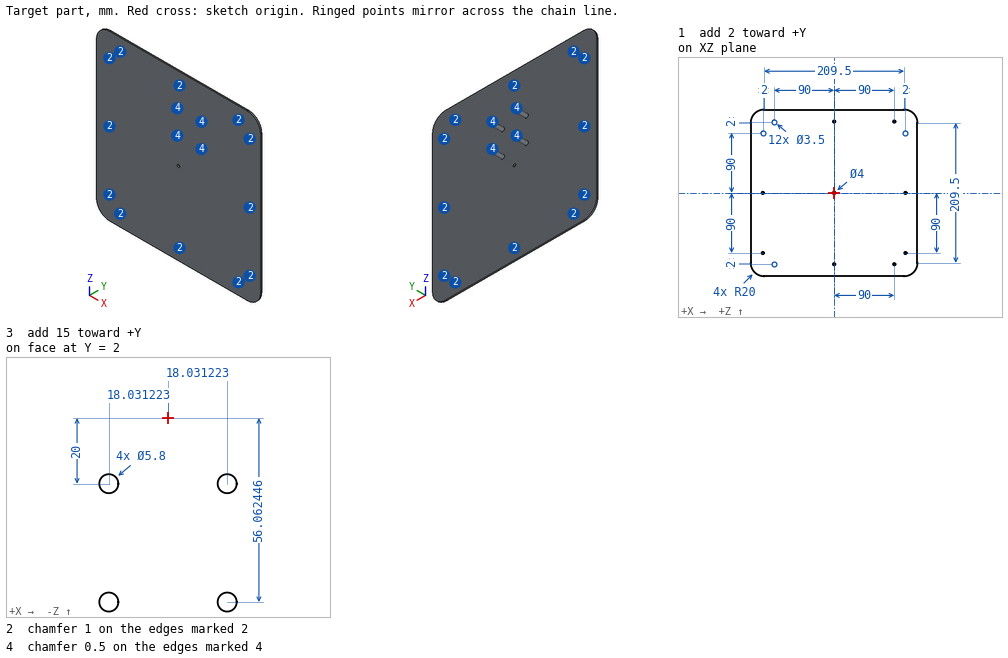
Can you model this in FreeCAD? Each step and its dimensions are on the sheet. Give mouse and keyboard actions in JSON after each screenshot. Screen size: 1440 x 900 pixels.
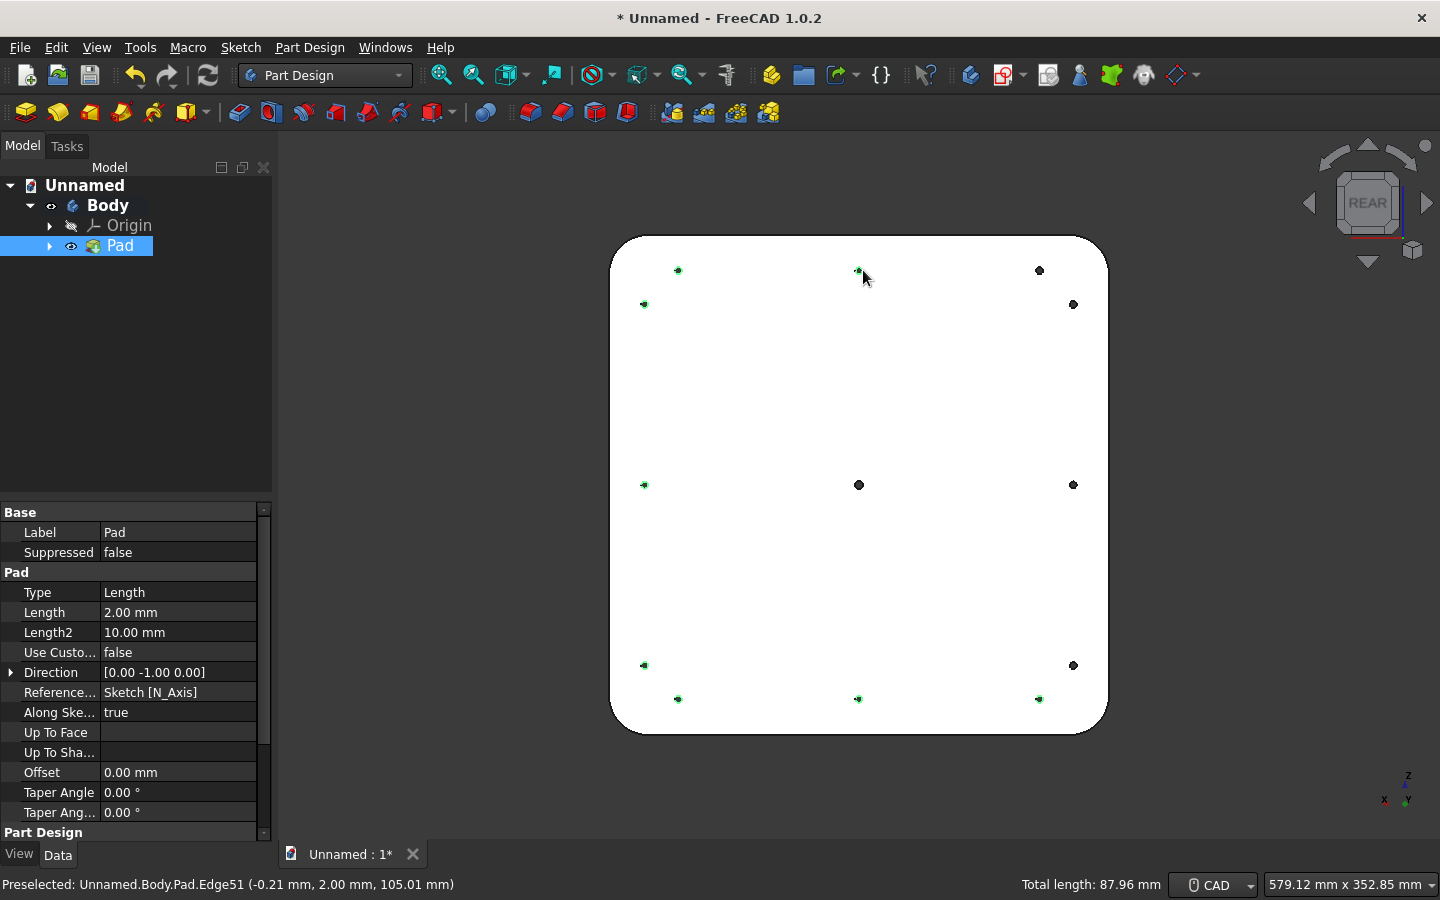
{"action": "left_click", "coordinate": [1043, 270], "text": "ctrl"}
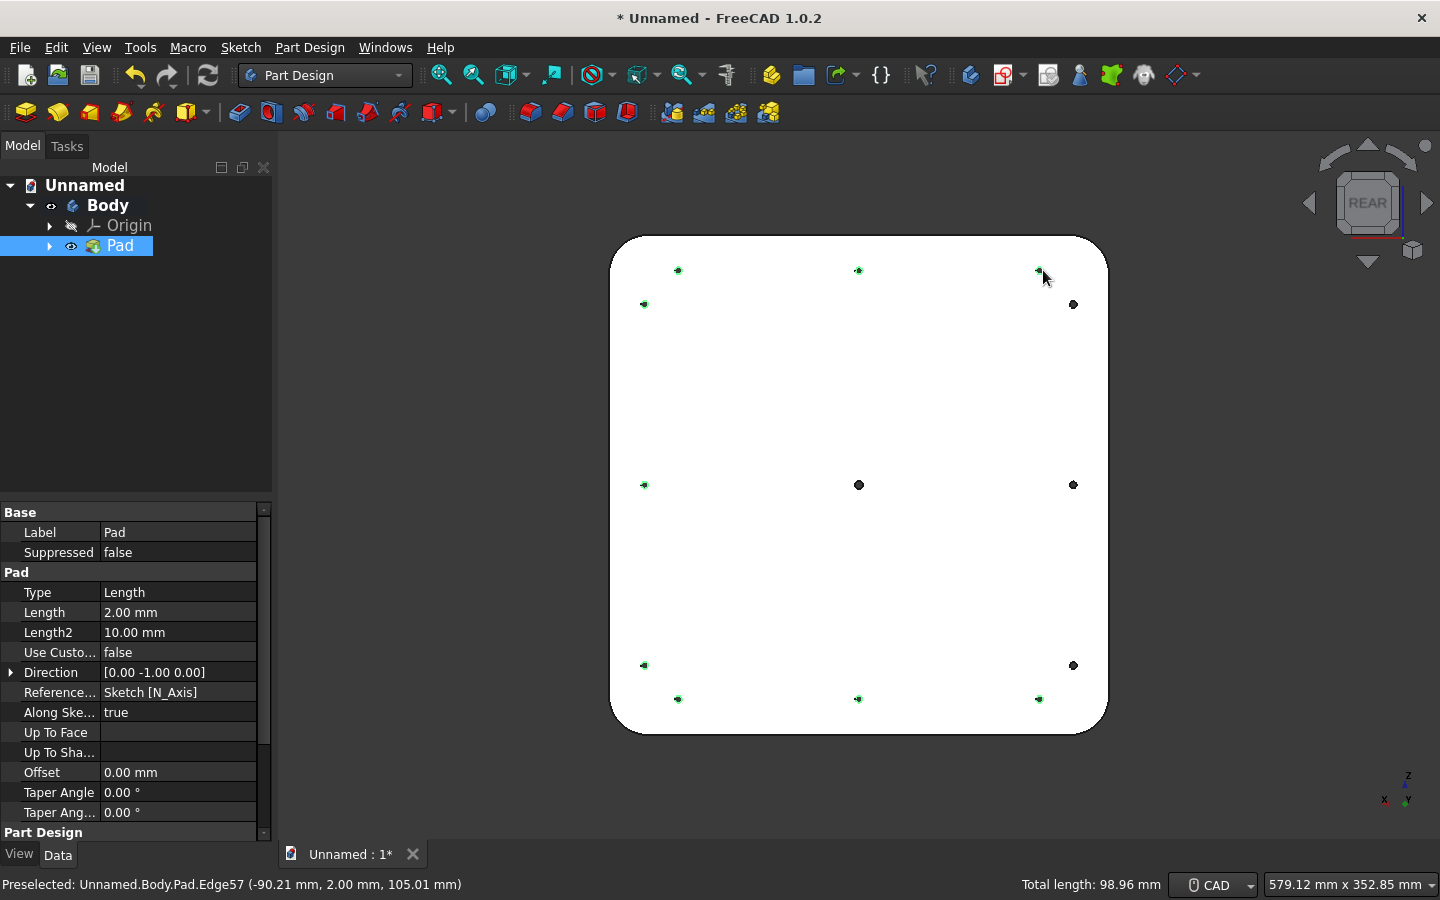
{"action": "left_click", "coordinate": [1077, 303], "text": "ctrl"}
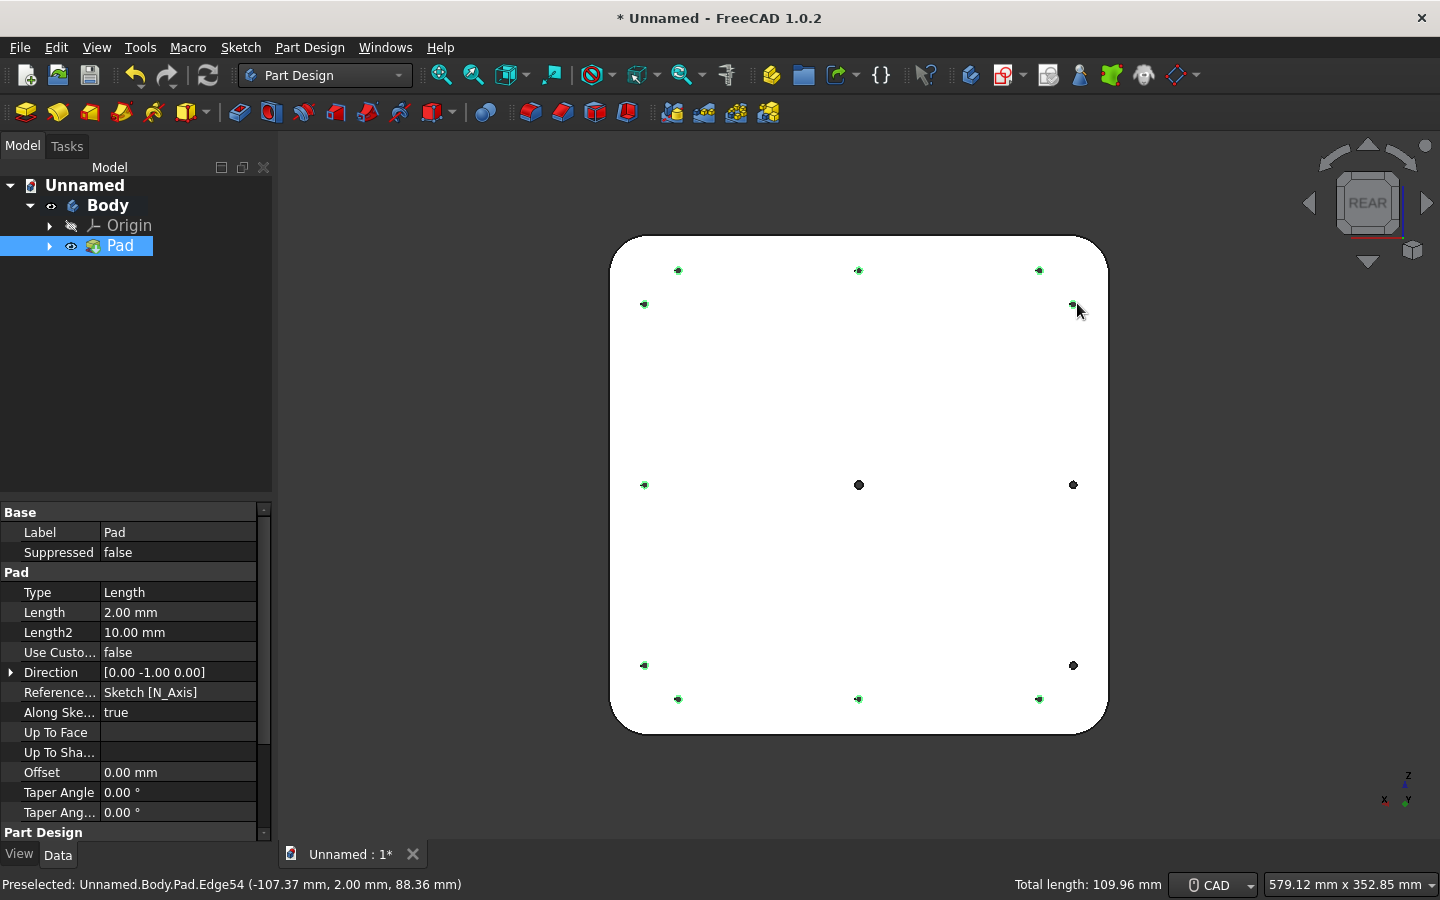
{"action": "left_click", "coordinate": [1077, 484], "text": "ctrl"}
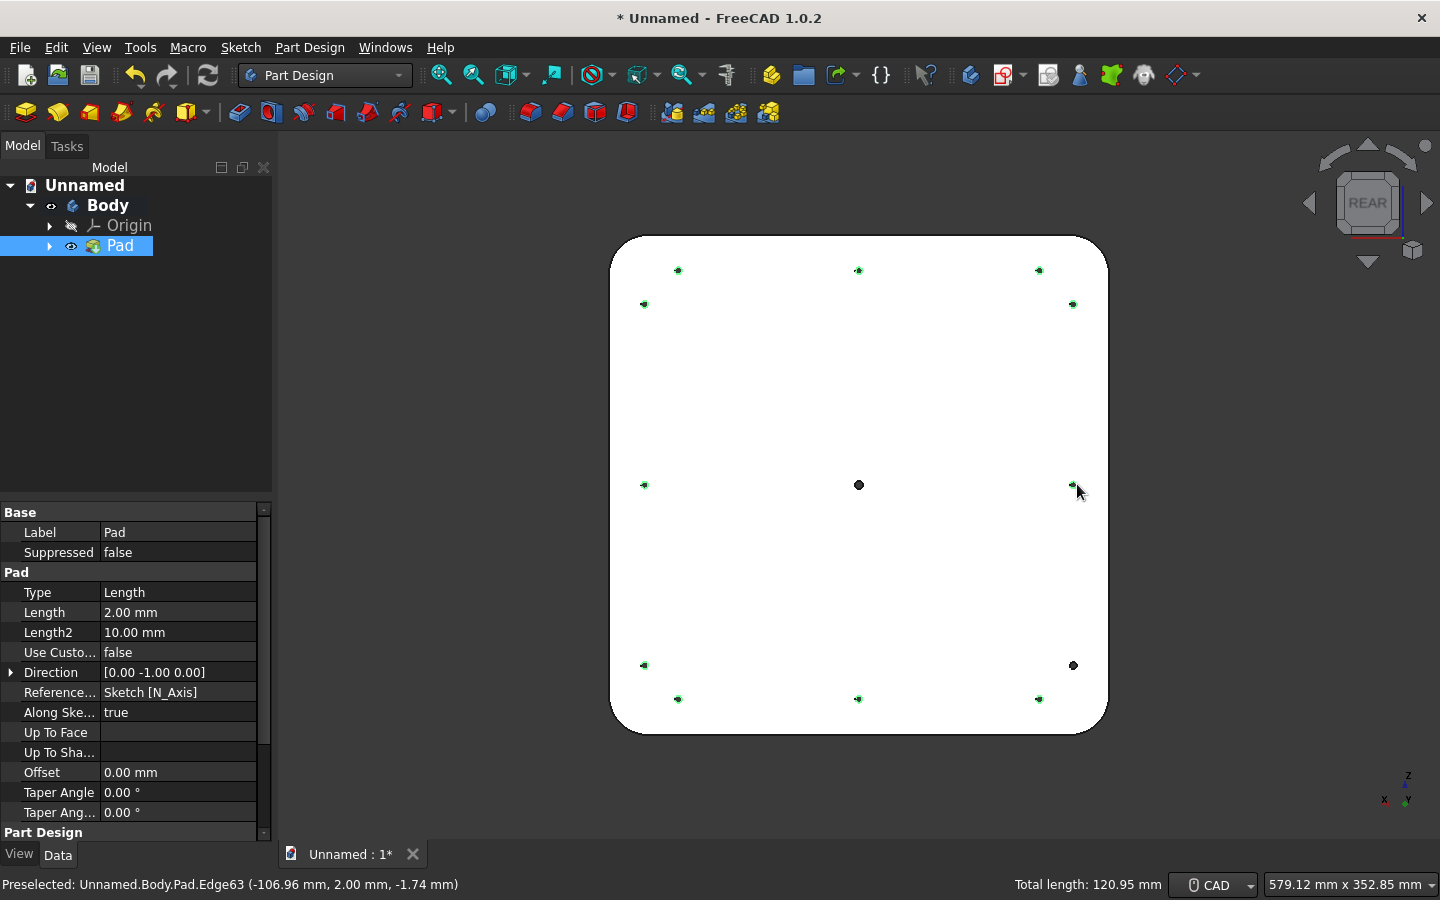
{"action": "left_click", "coordinate": [1077, 665], "text": "ctrl"}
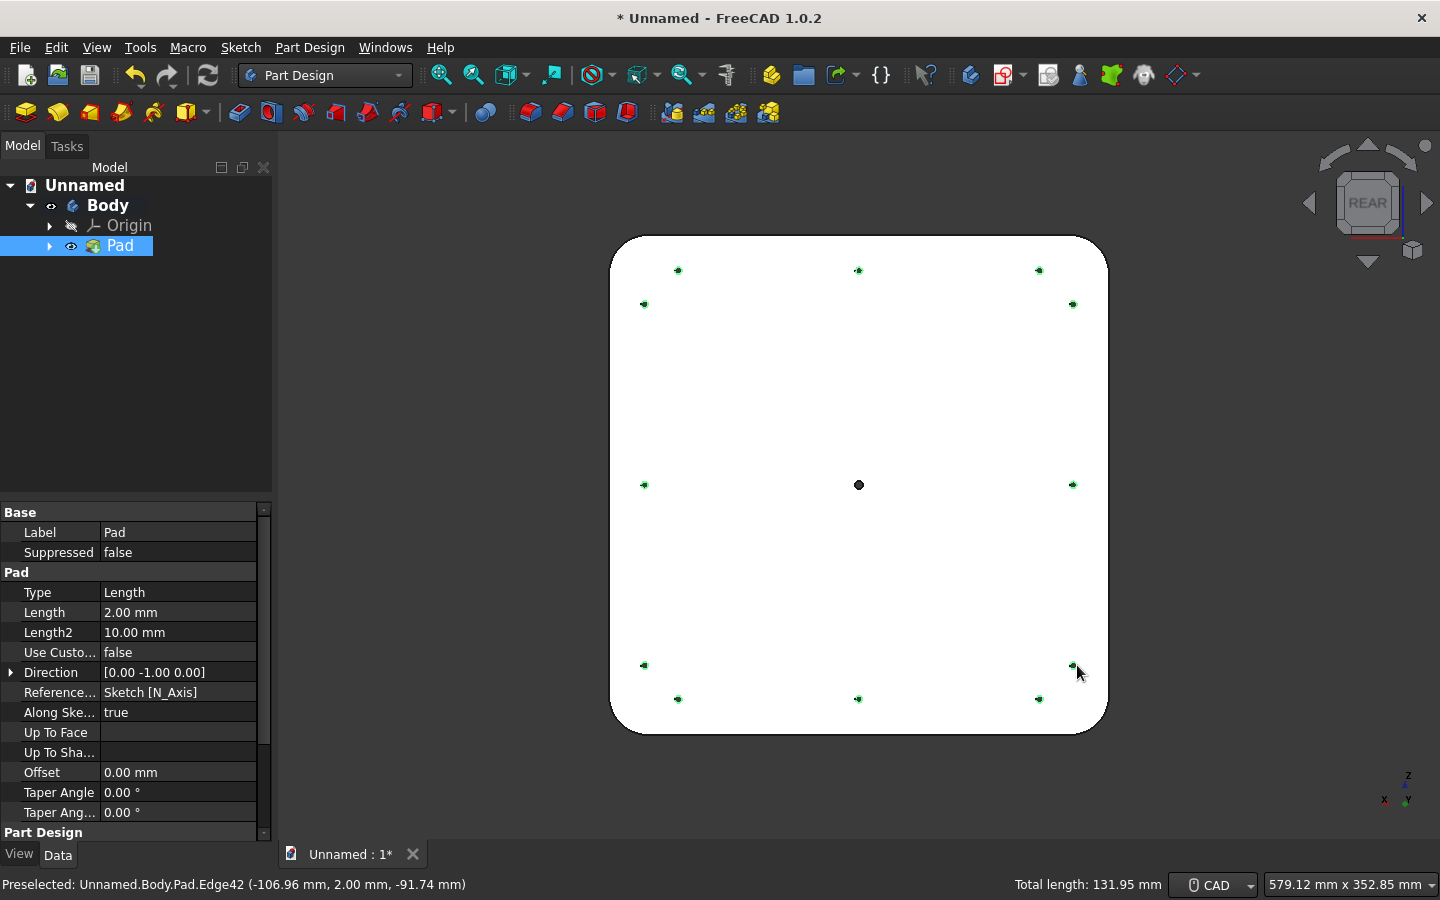
{"action": "left_click", "coordinate": [564, 112]}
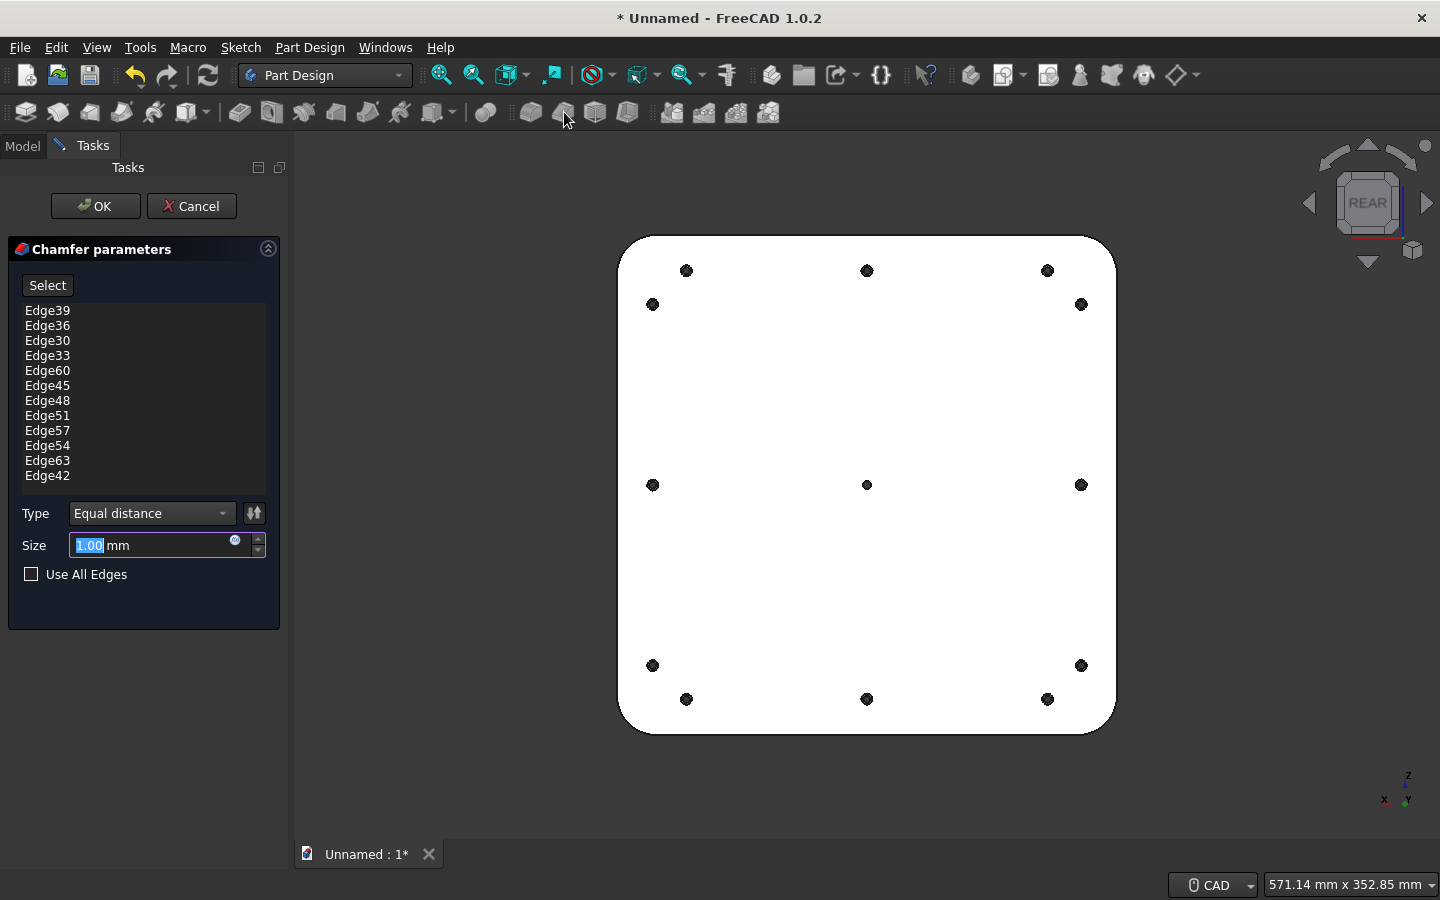
{"action": "type", "text": "1"}
{"action": "key", "text": "Tab"}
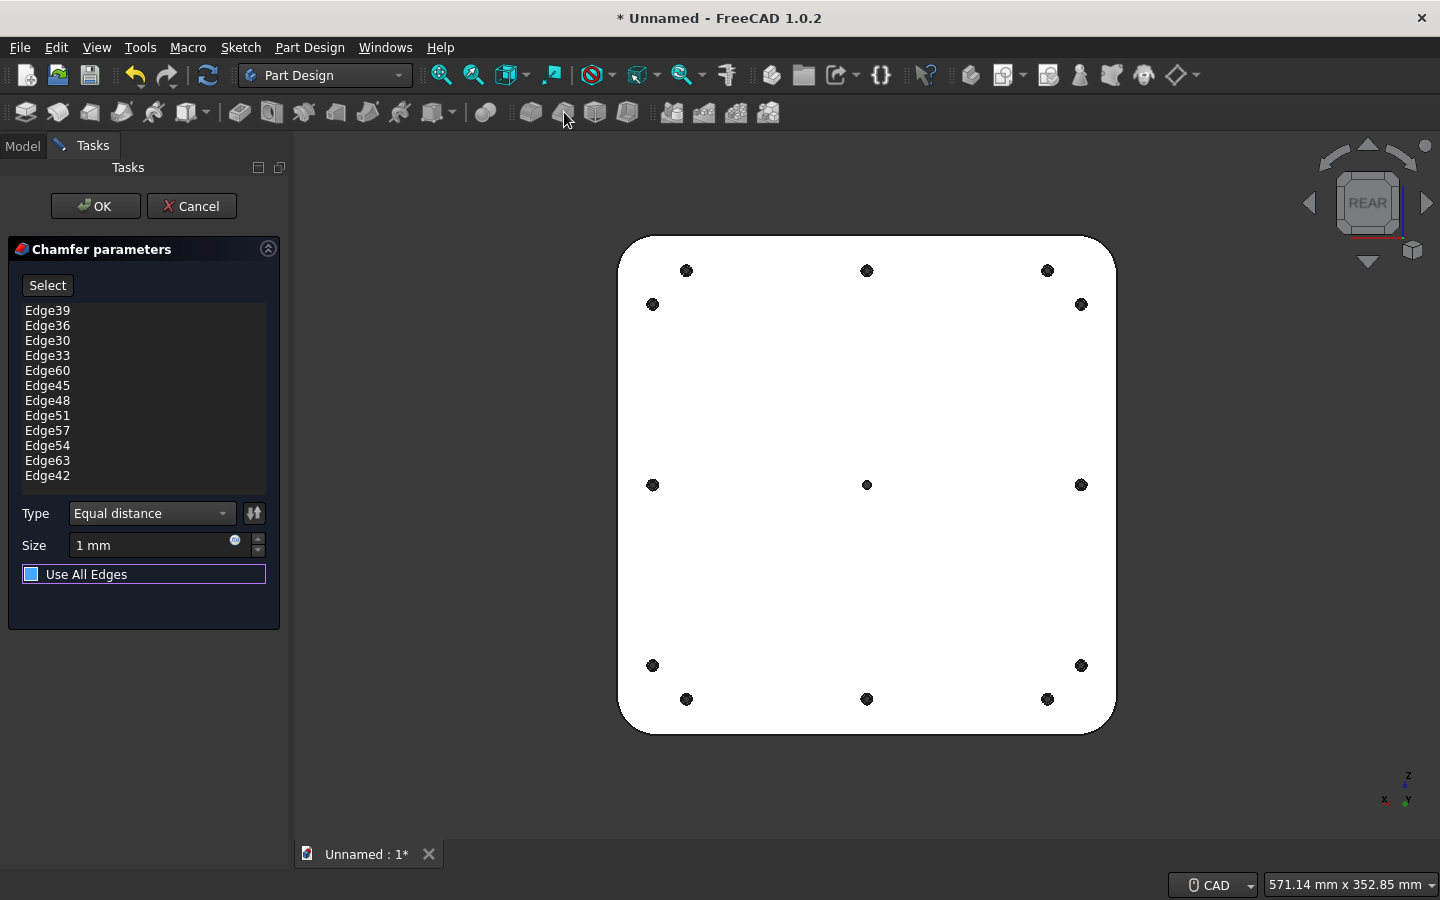
{"action": "left_click", "coordinate": [96, 206]}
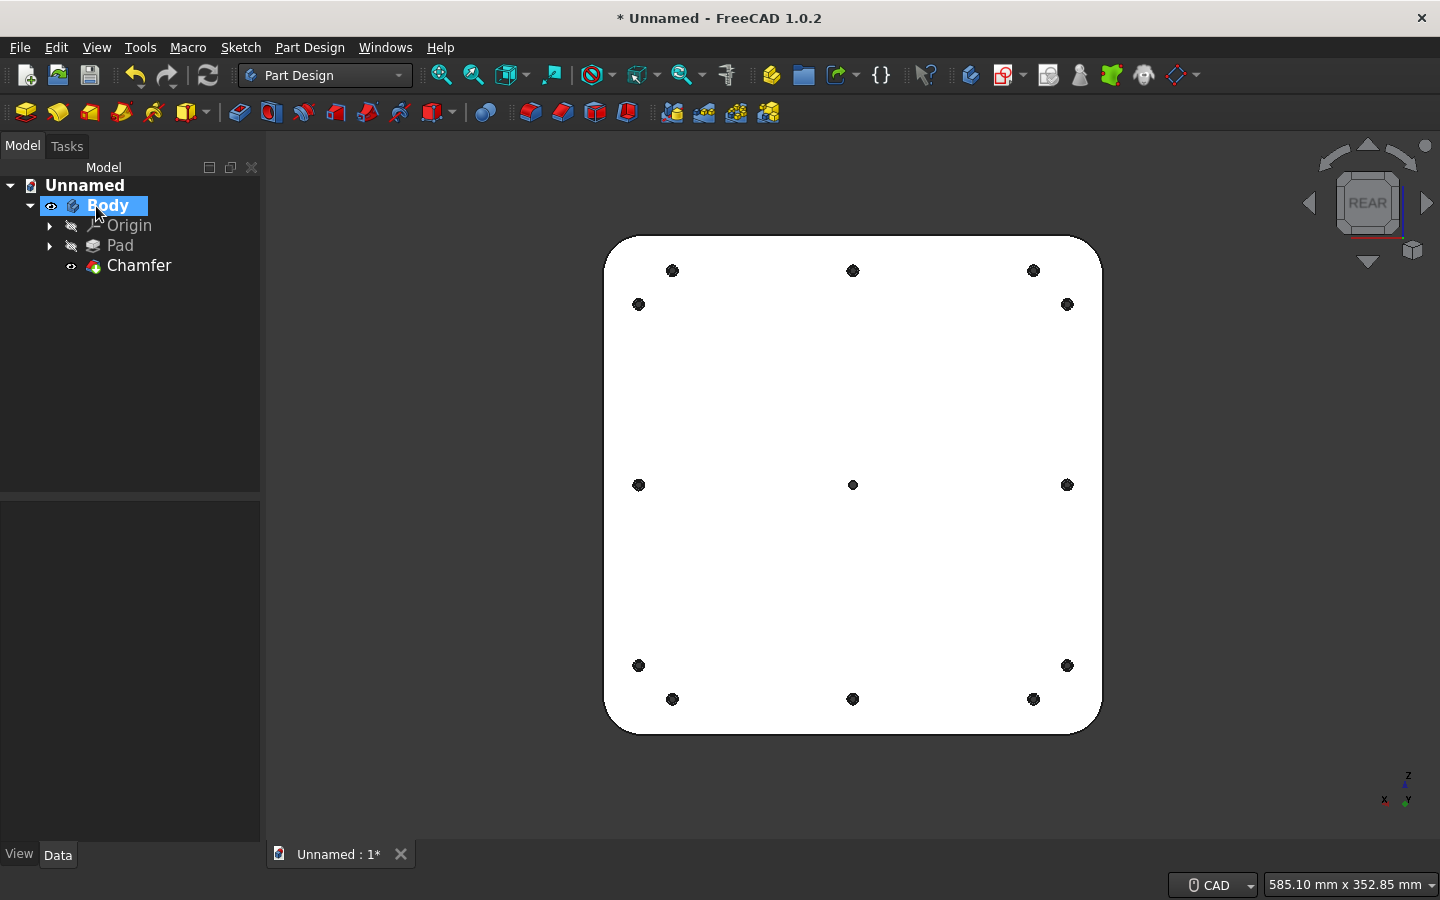
{"action": "left_click", "coordinate": [781, 412]}